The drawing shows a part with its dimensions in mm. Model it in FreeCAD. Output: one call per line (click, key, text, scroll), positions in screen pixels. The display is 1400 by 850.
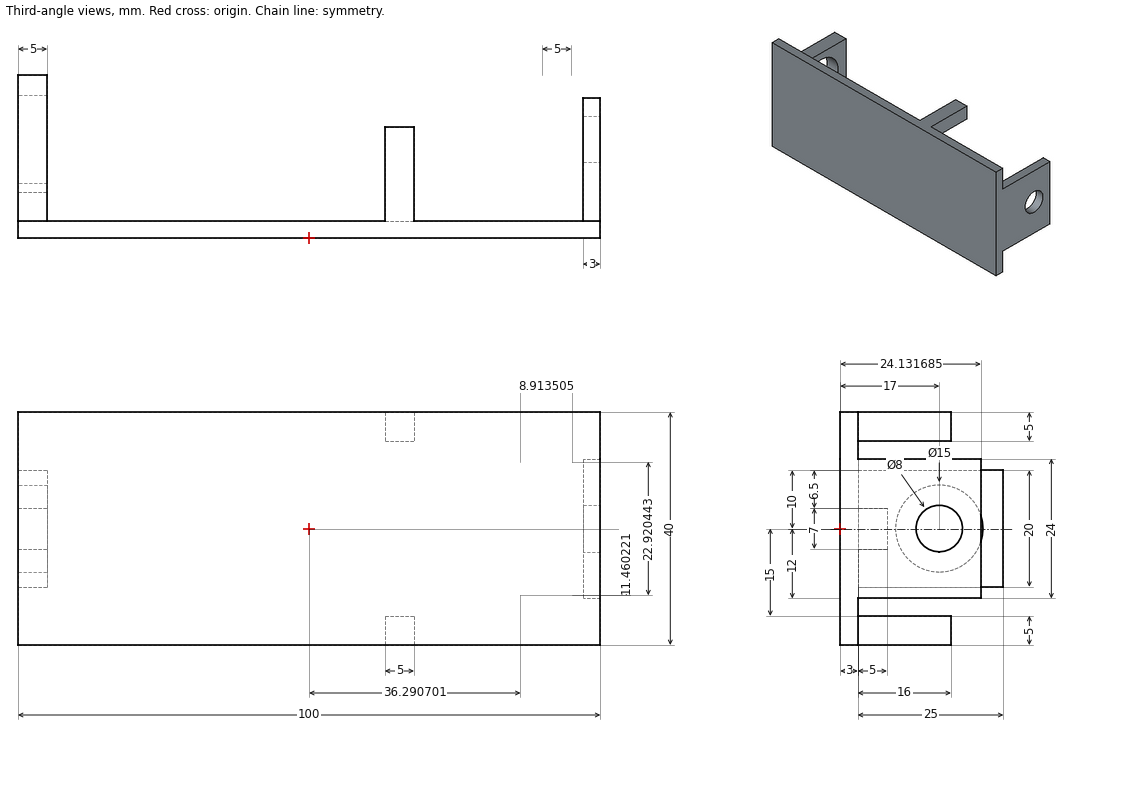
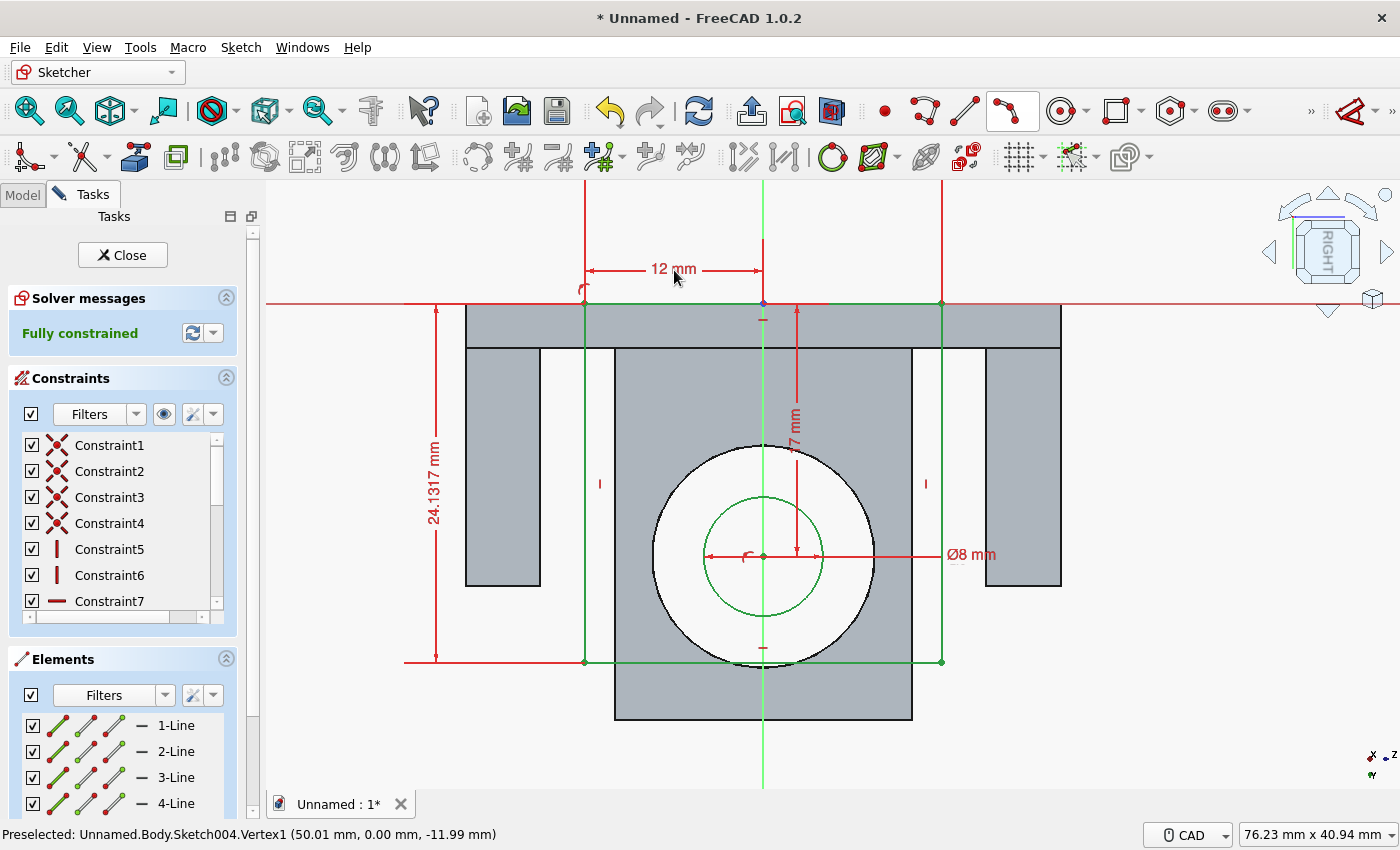
click(123, 255)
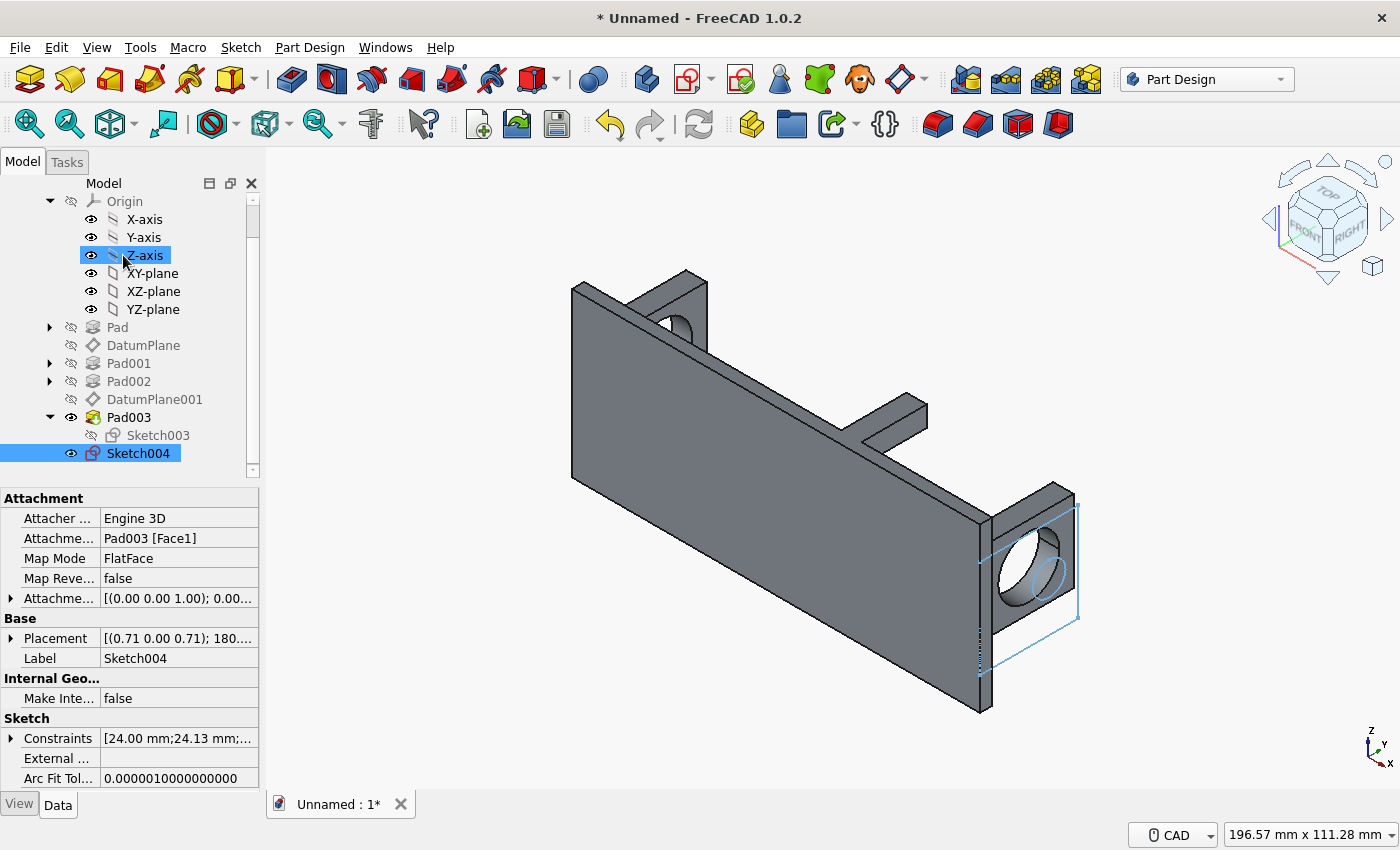
click(30, 80)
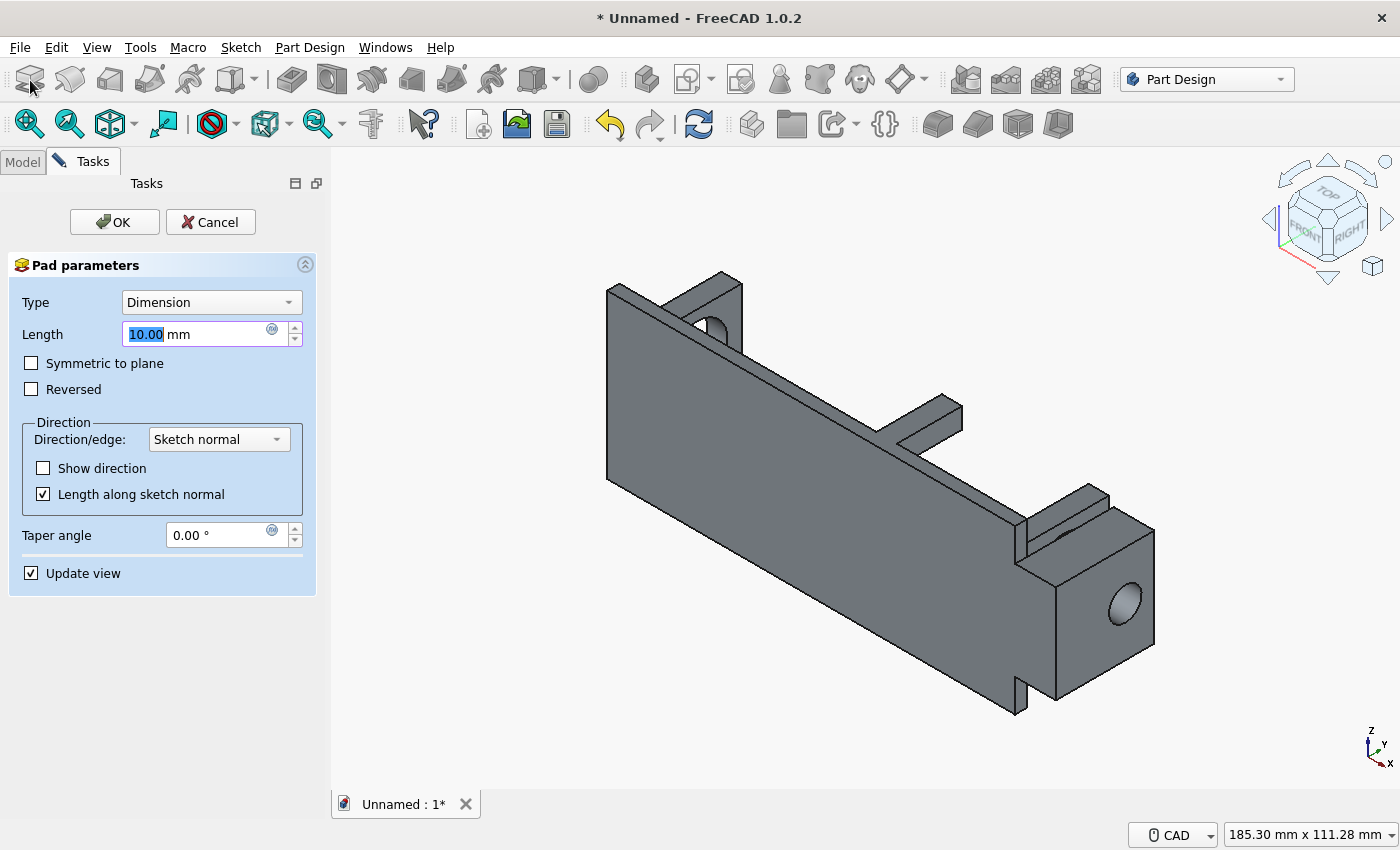
text(3)
key(Tab)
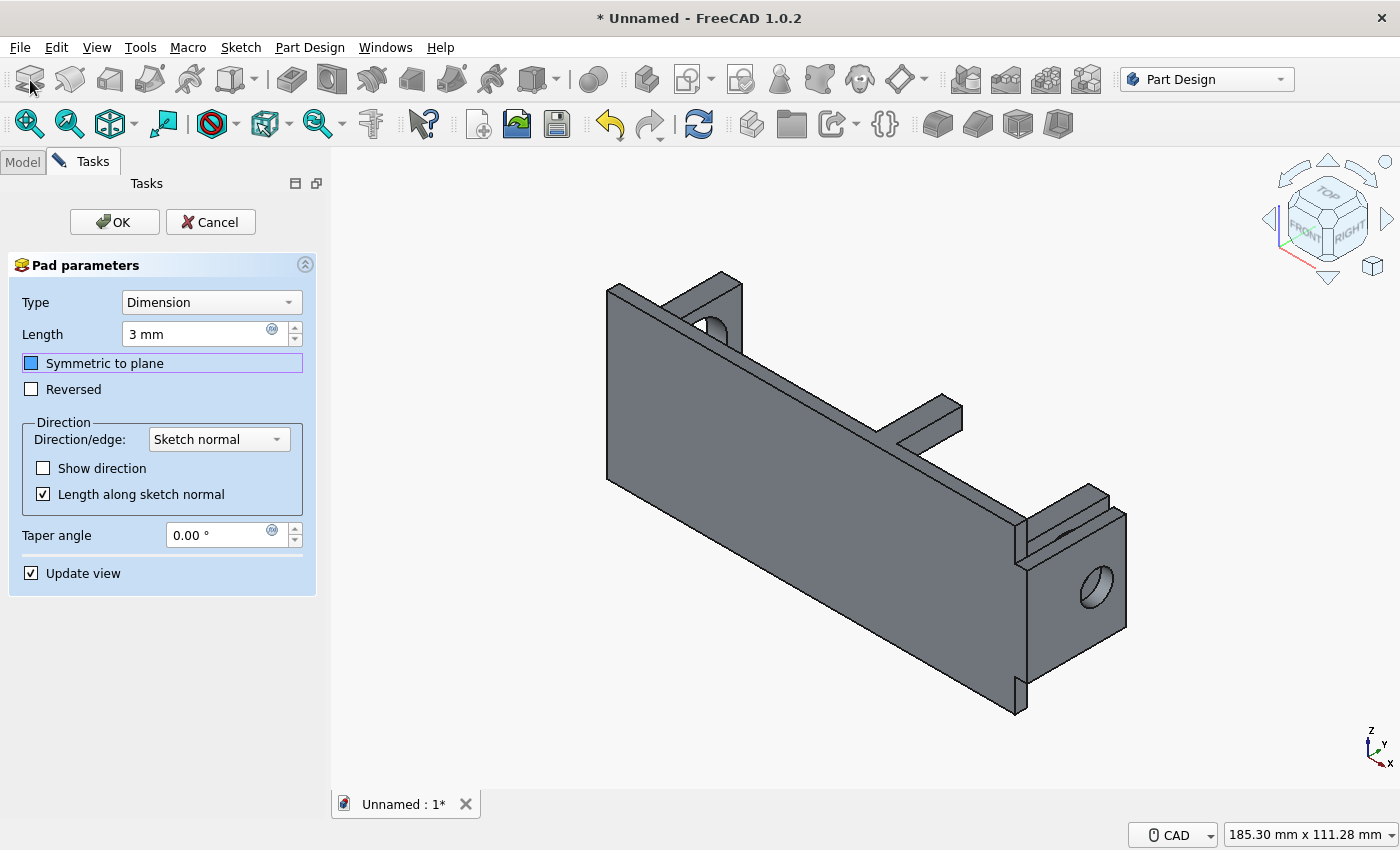
click(30, 389)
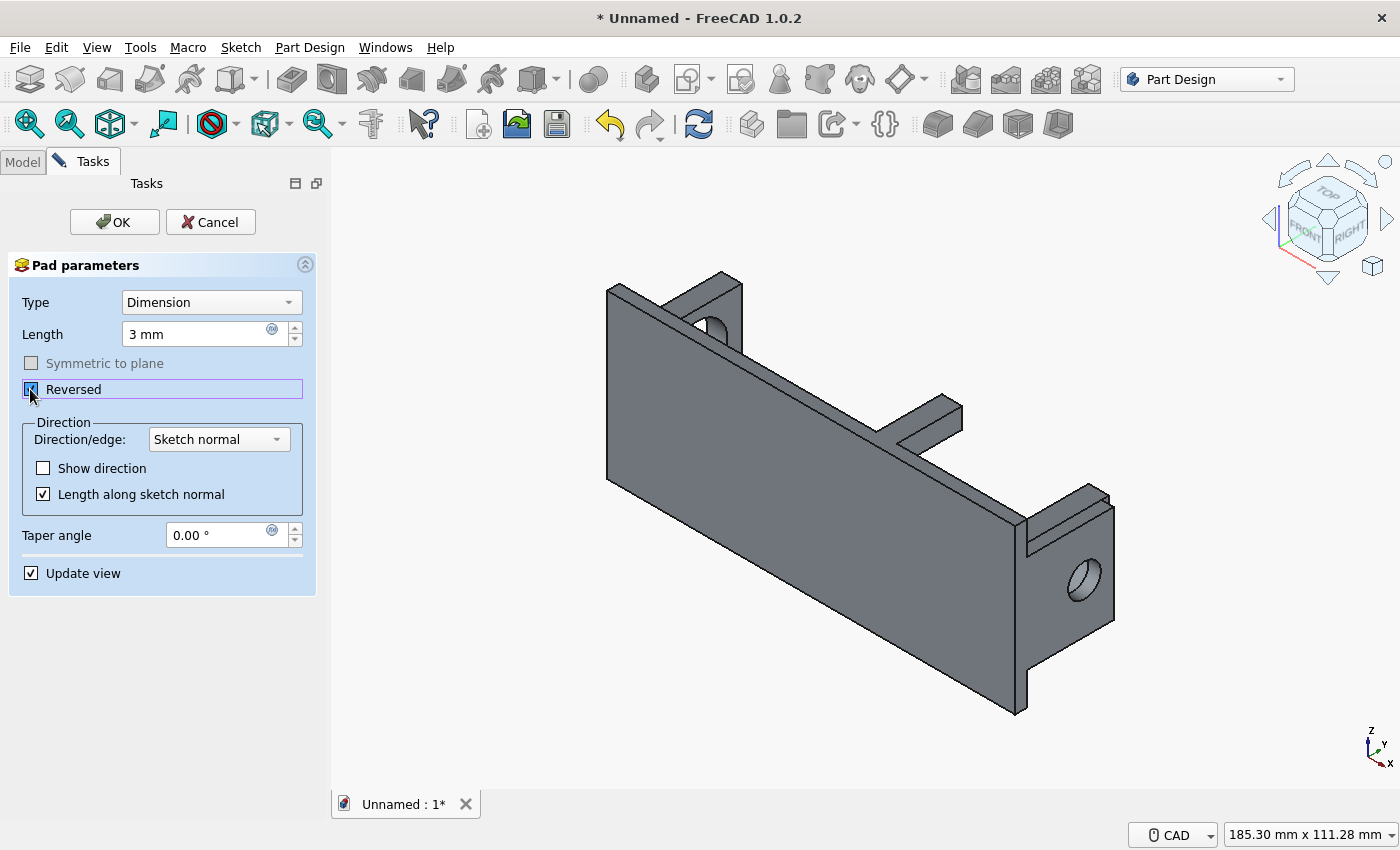
click(115, 222)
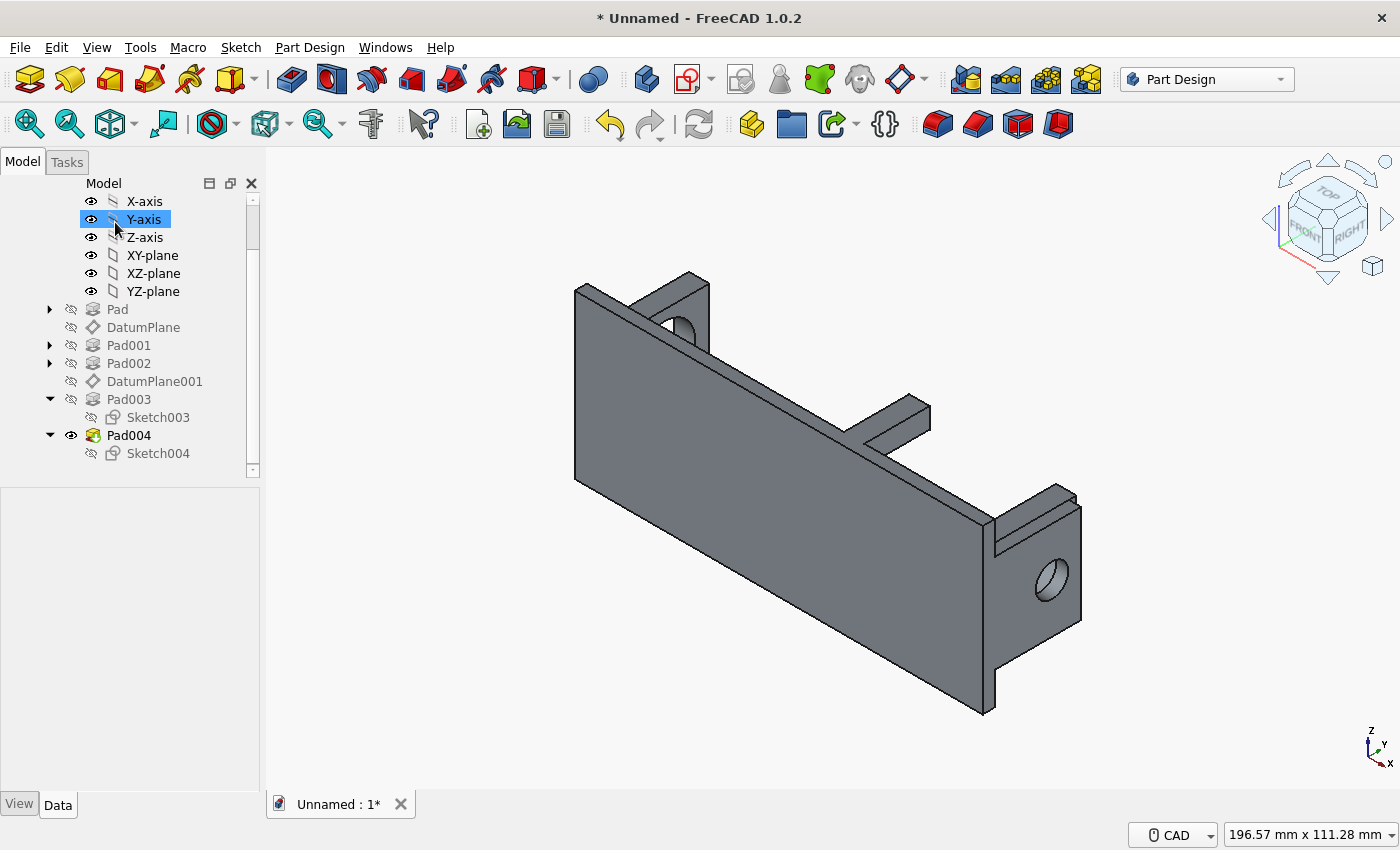
key(4)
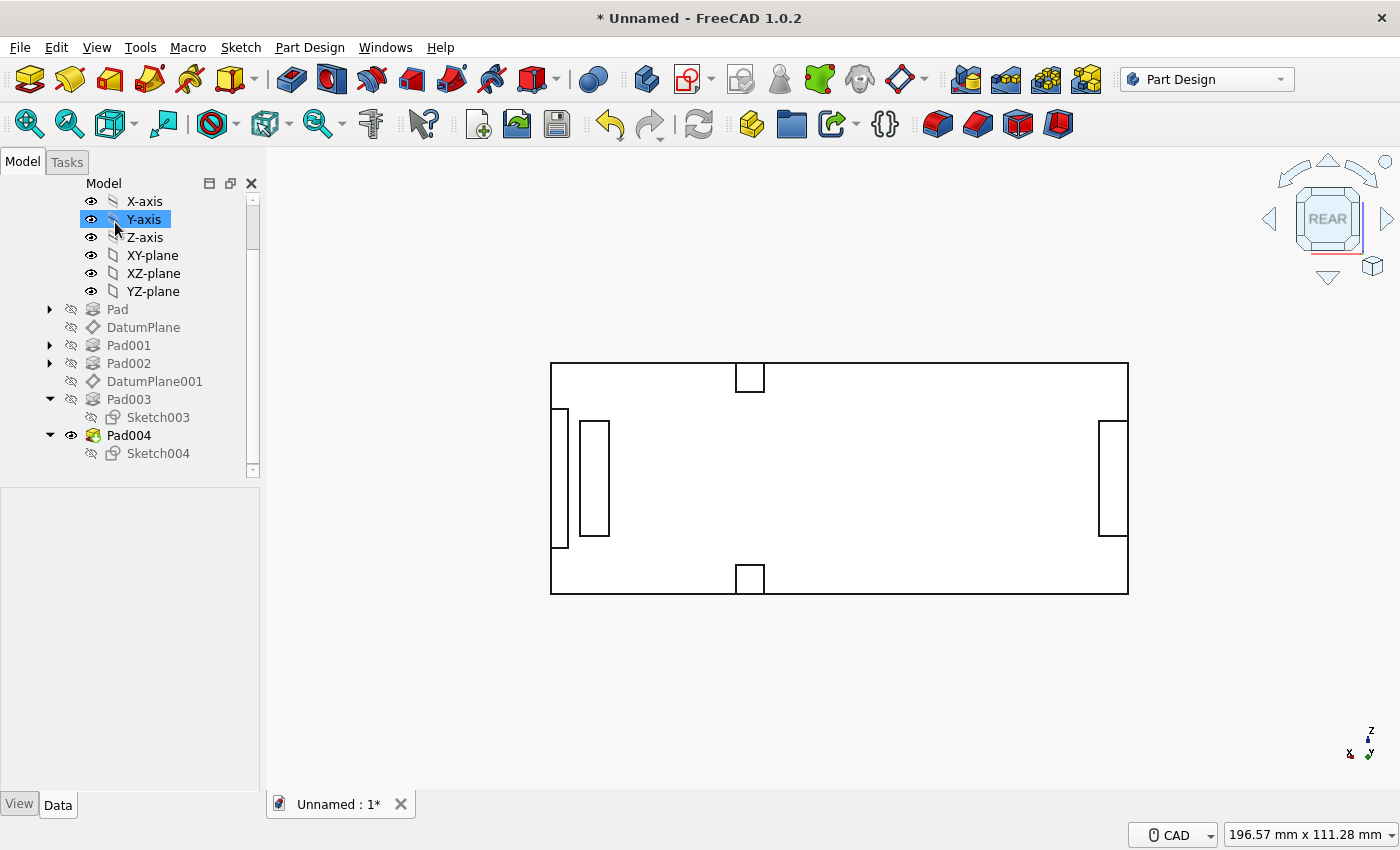
click(922, 477)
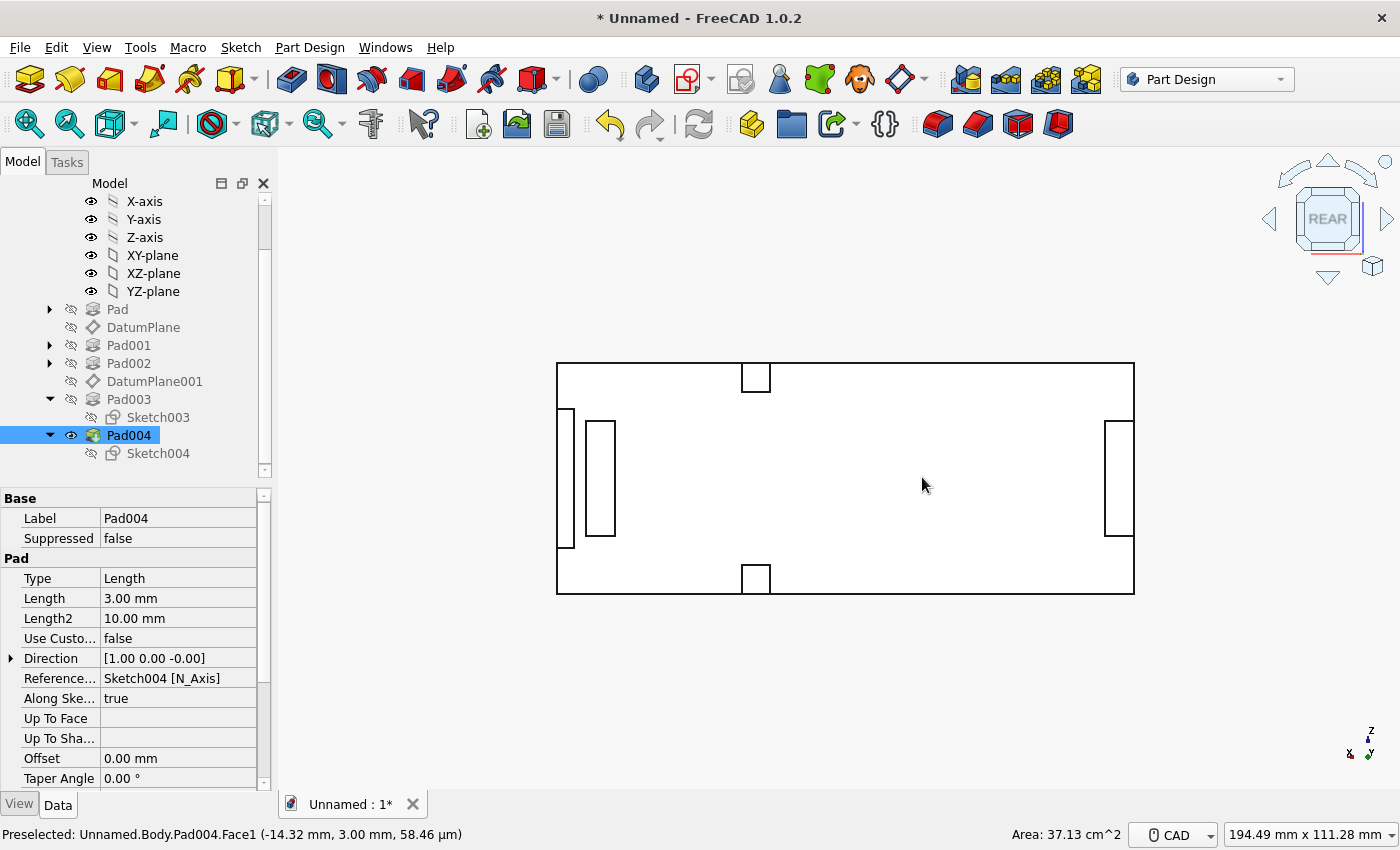
click(688, 80)